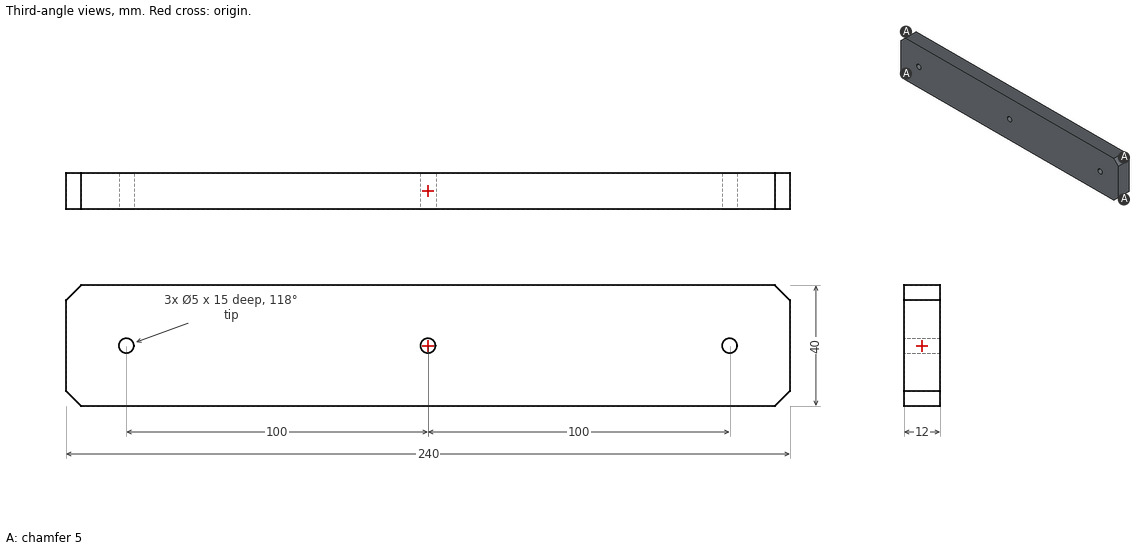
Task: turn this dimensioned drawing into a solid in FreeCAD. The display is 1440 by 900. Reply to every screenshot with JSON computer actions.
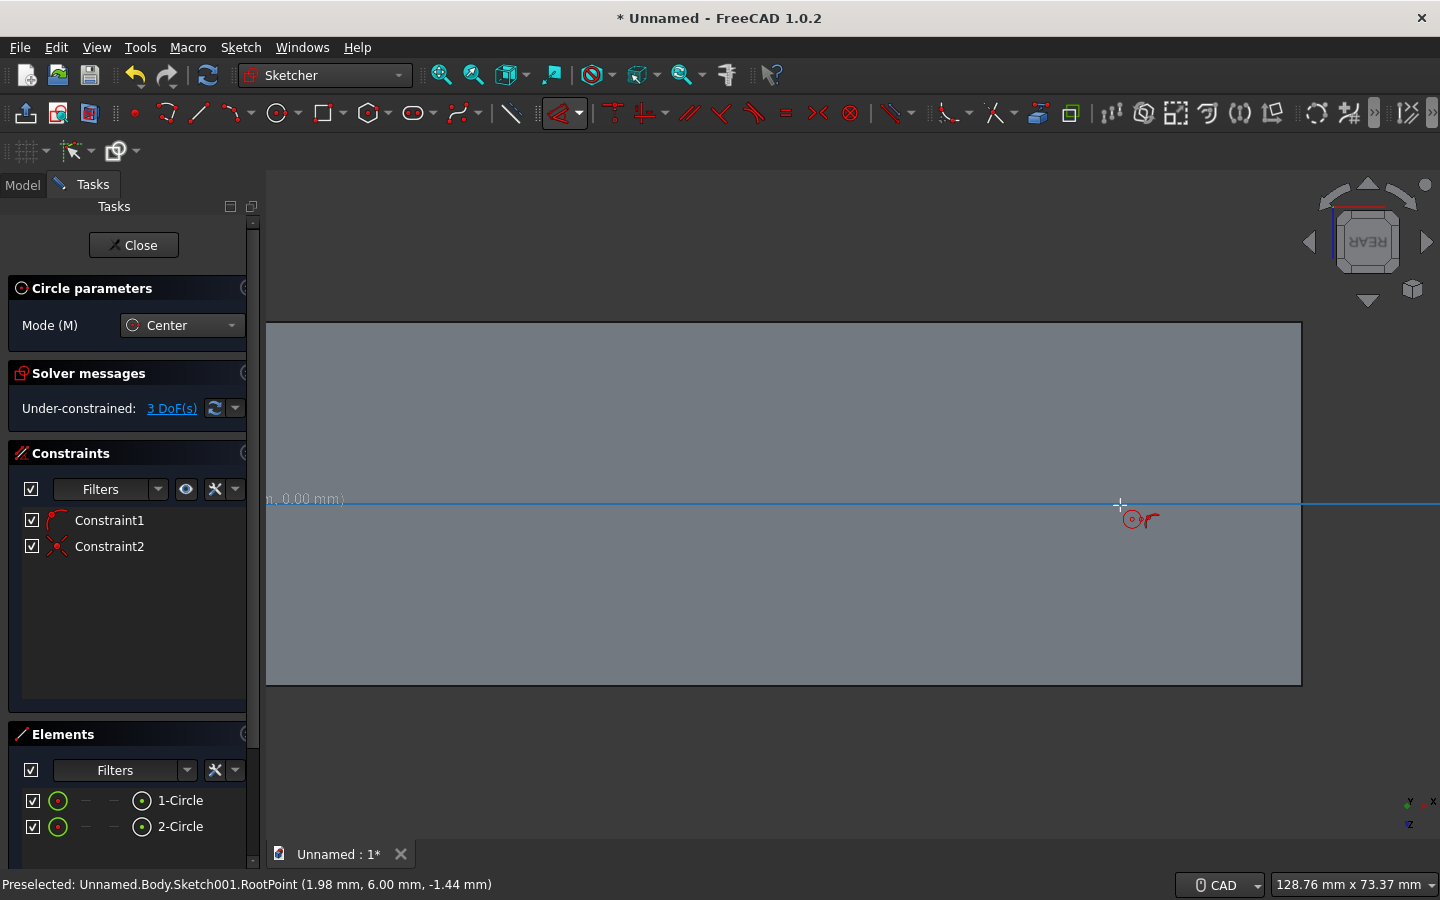
{"action": "left_click", "coordinate": [1119, 504]}
{"action": "left_click", "coordinate": [1135, 488]}
{"action": "key", "text": "Escape"}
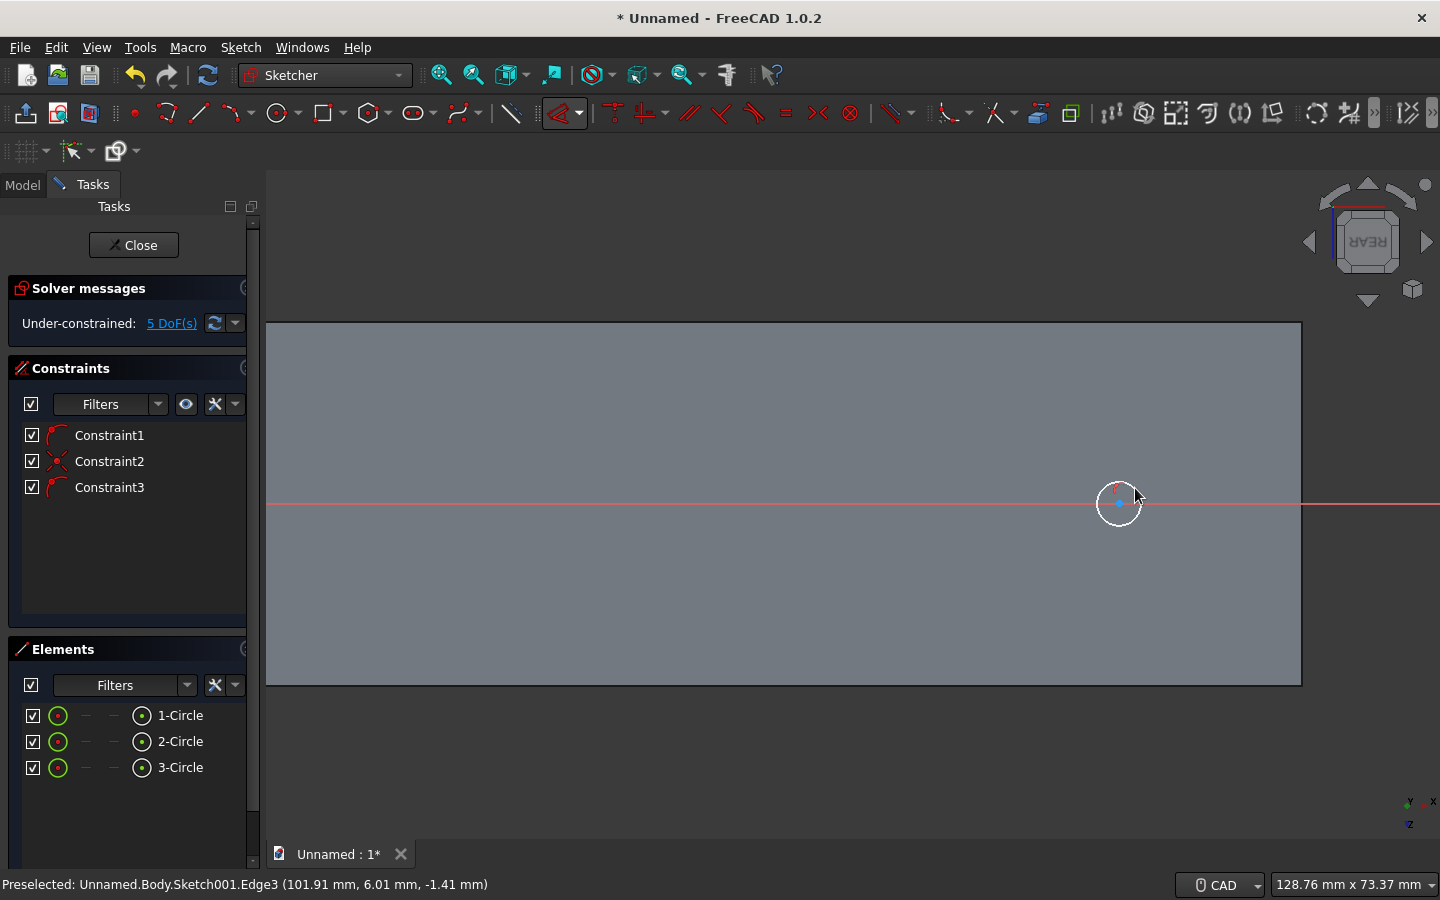
{"action": "scroll", "coordinate": [1120, 505], "scroll_direction": "down", "scroll_amount": 5}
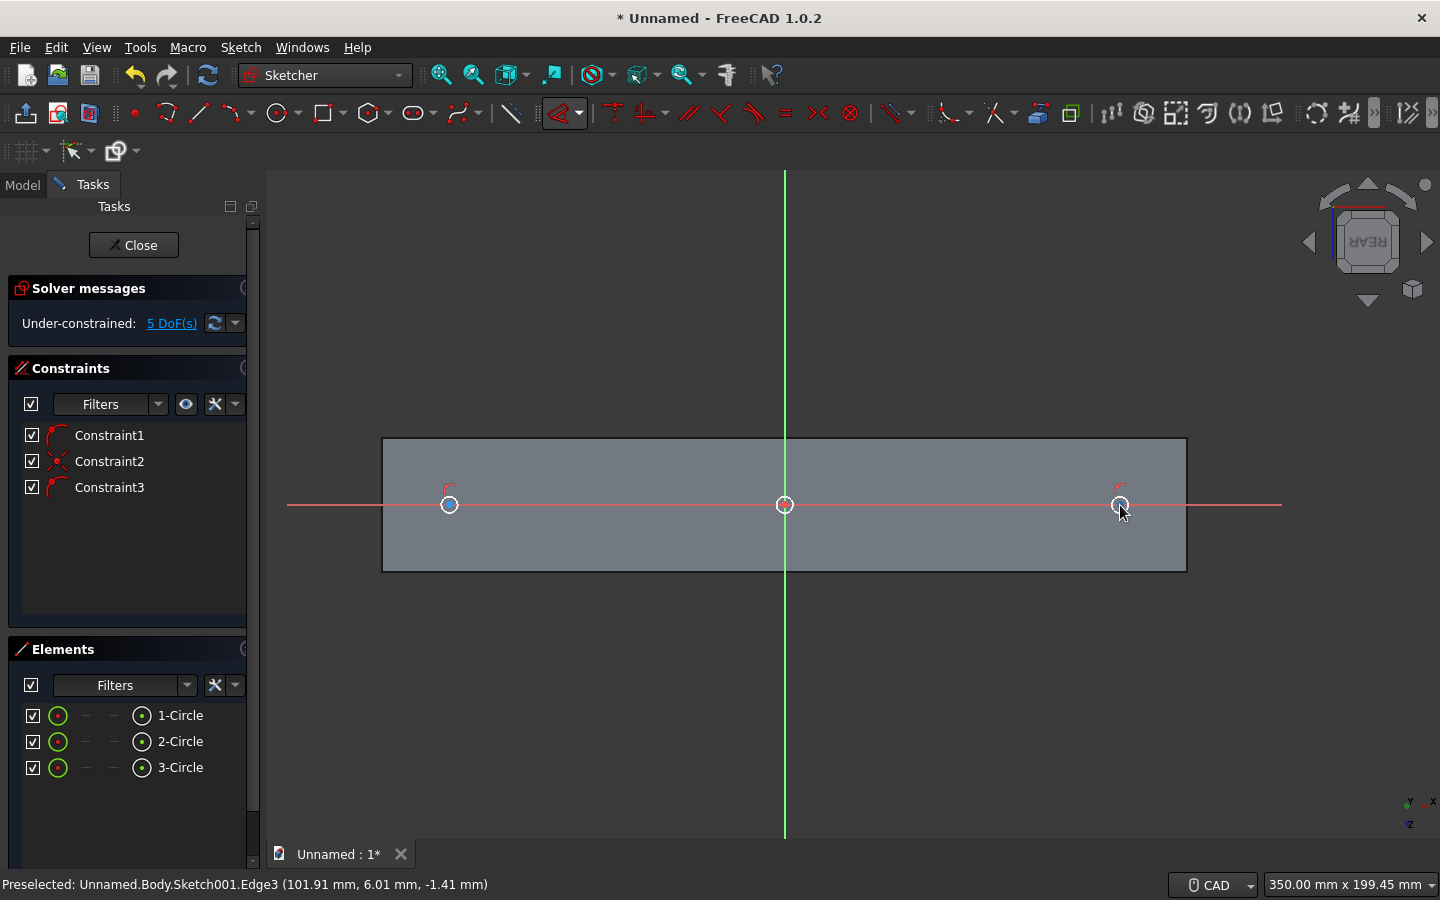
{"action": "scroll", "coordinate": [455, 499], "scroll_direction": "up", "scroll_amount": 5}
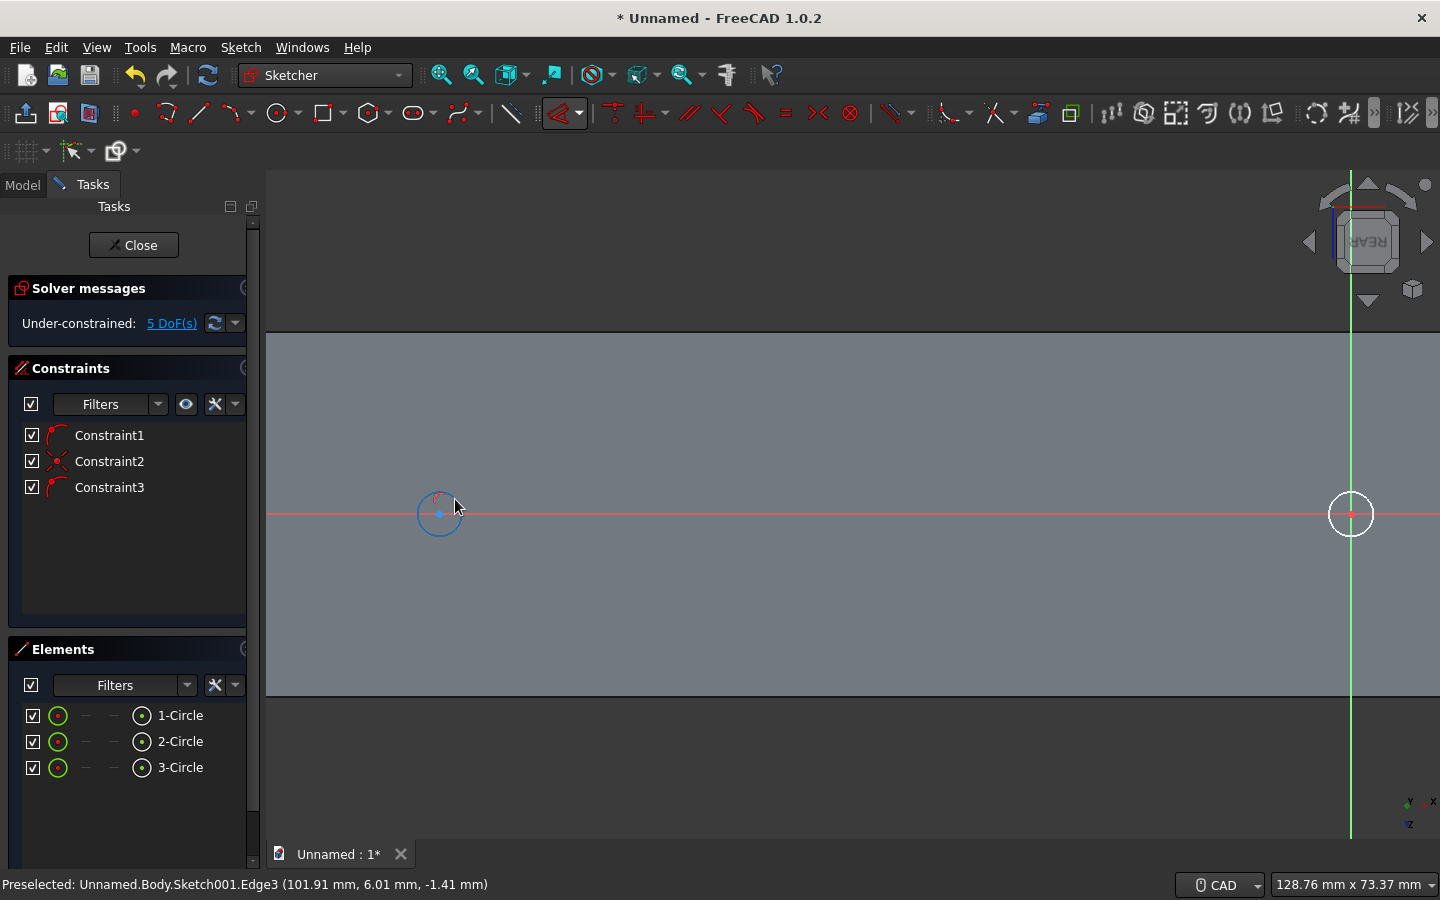
{"action": "left_click", "coordinate": [455, 499]}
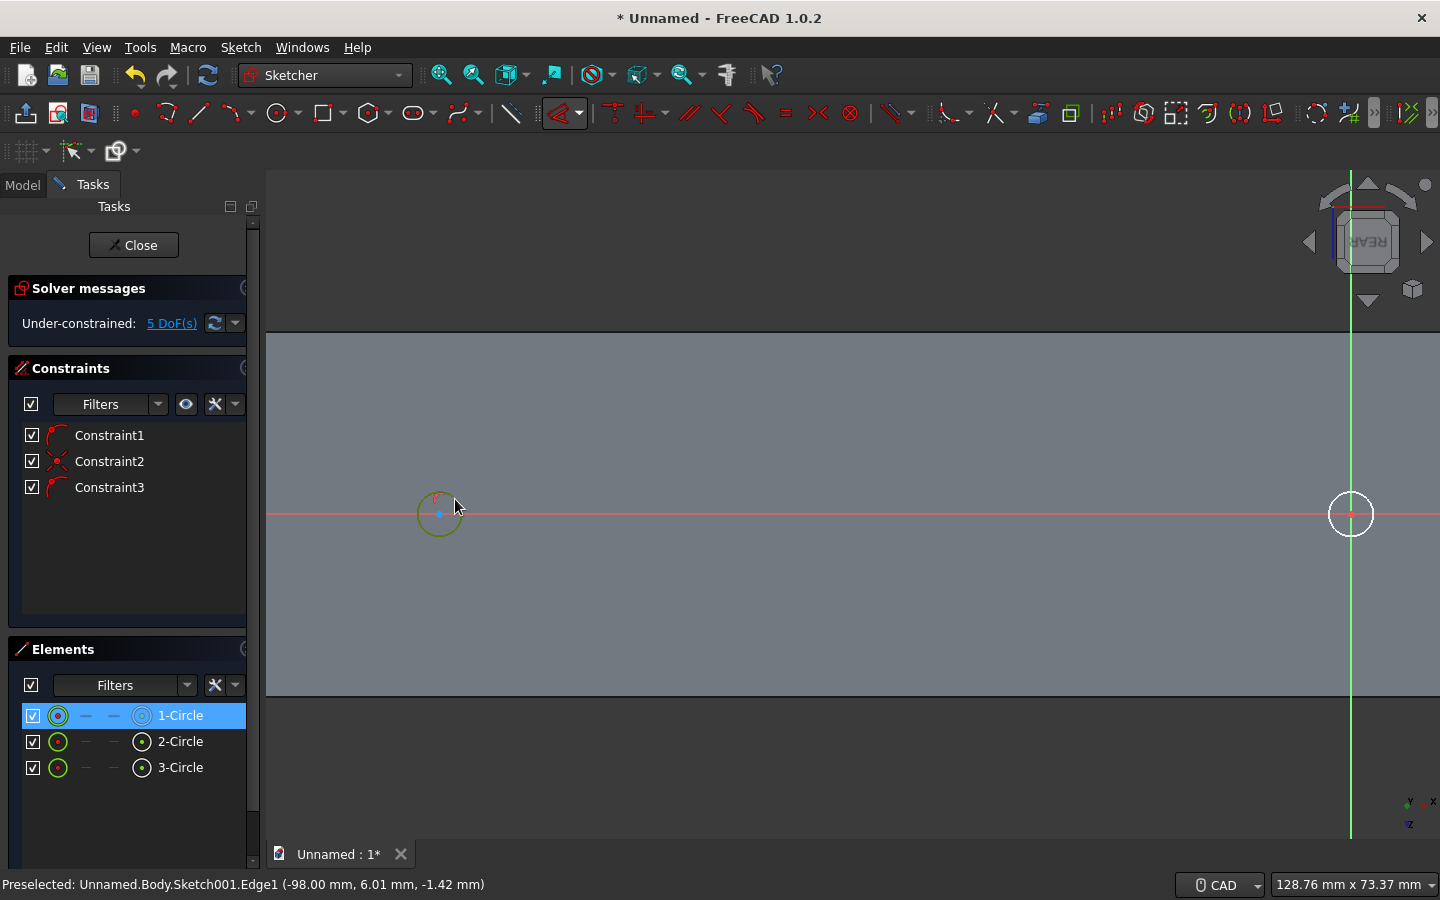
{"action": "scroll", "coordinate": [455, 499], "scroll_direction": "down", "scroll_amount": 5}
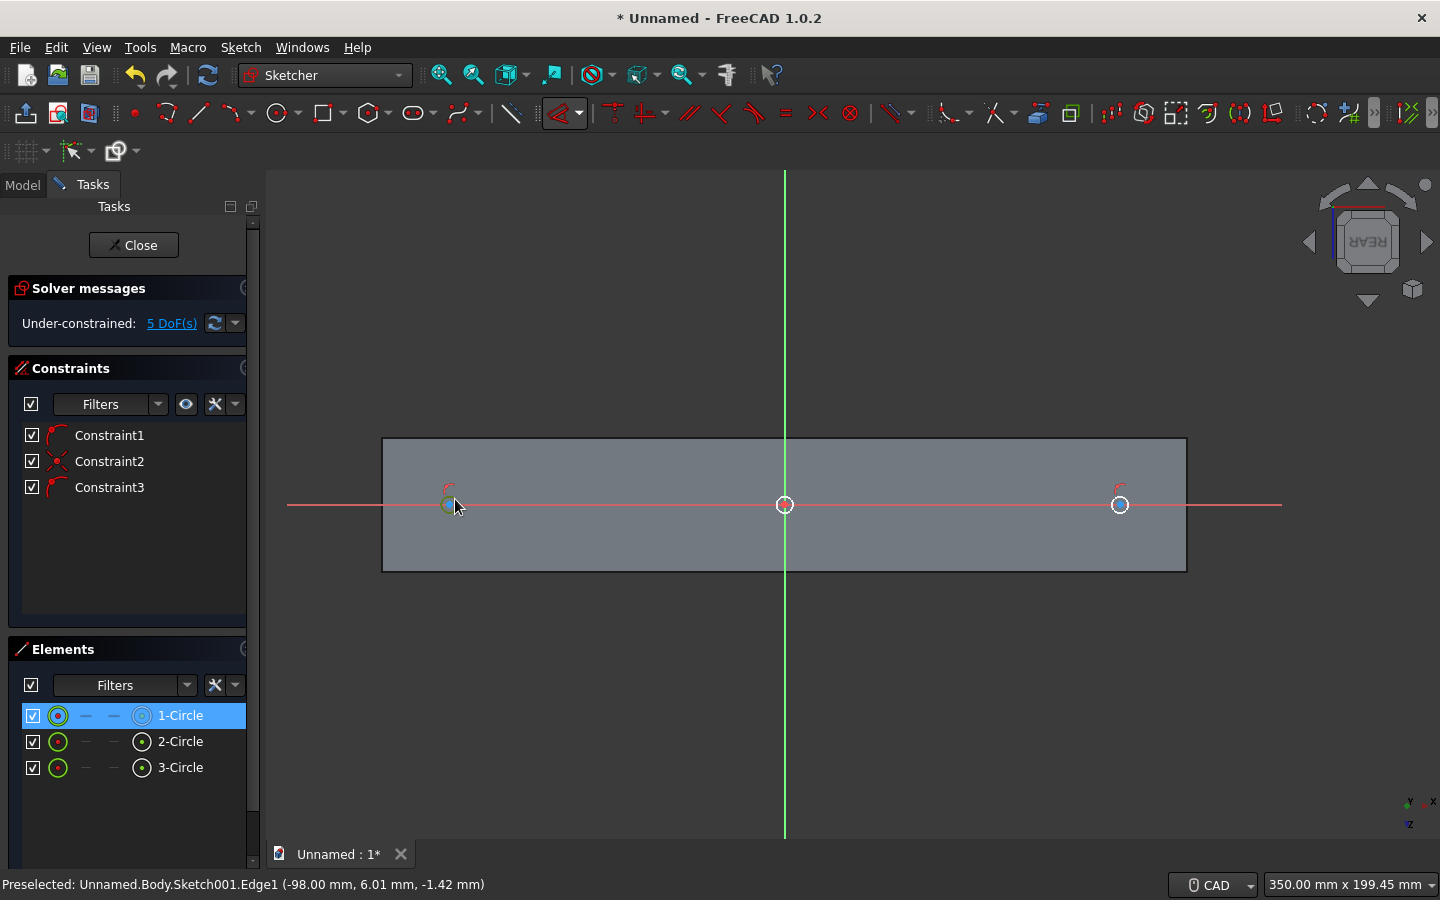
{"action": "scroll", "coordinate": [791, 499], "scroll_direction": "up", "scroll_amount": 5}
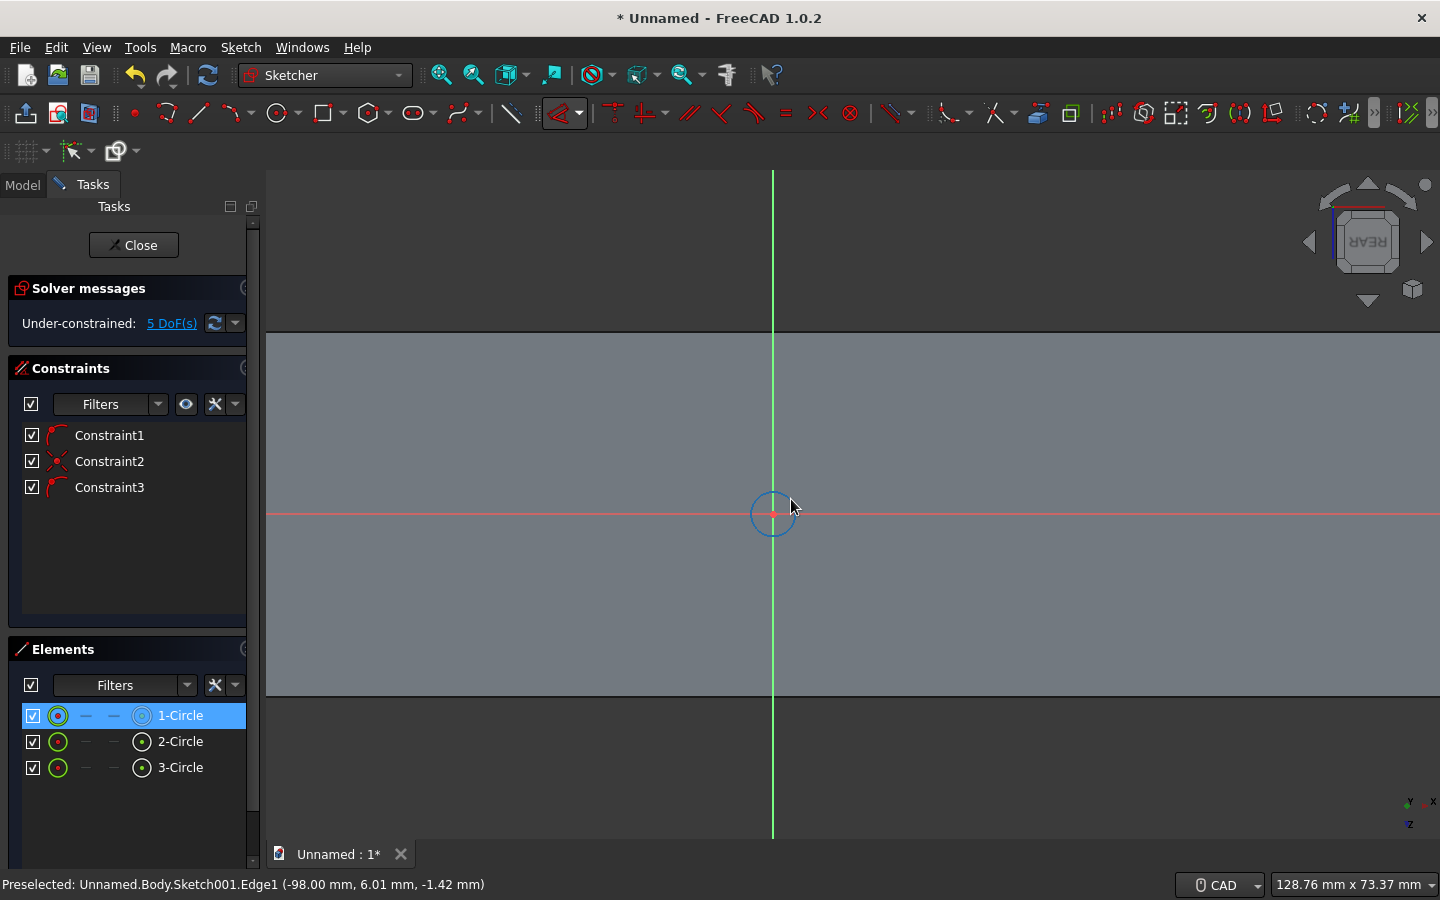
{"action": "left_click", "coordinate": [789, 499]}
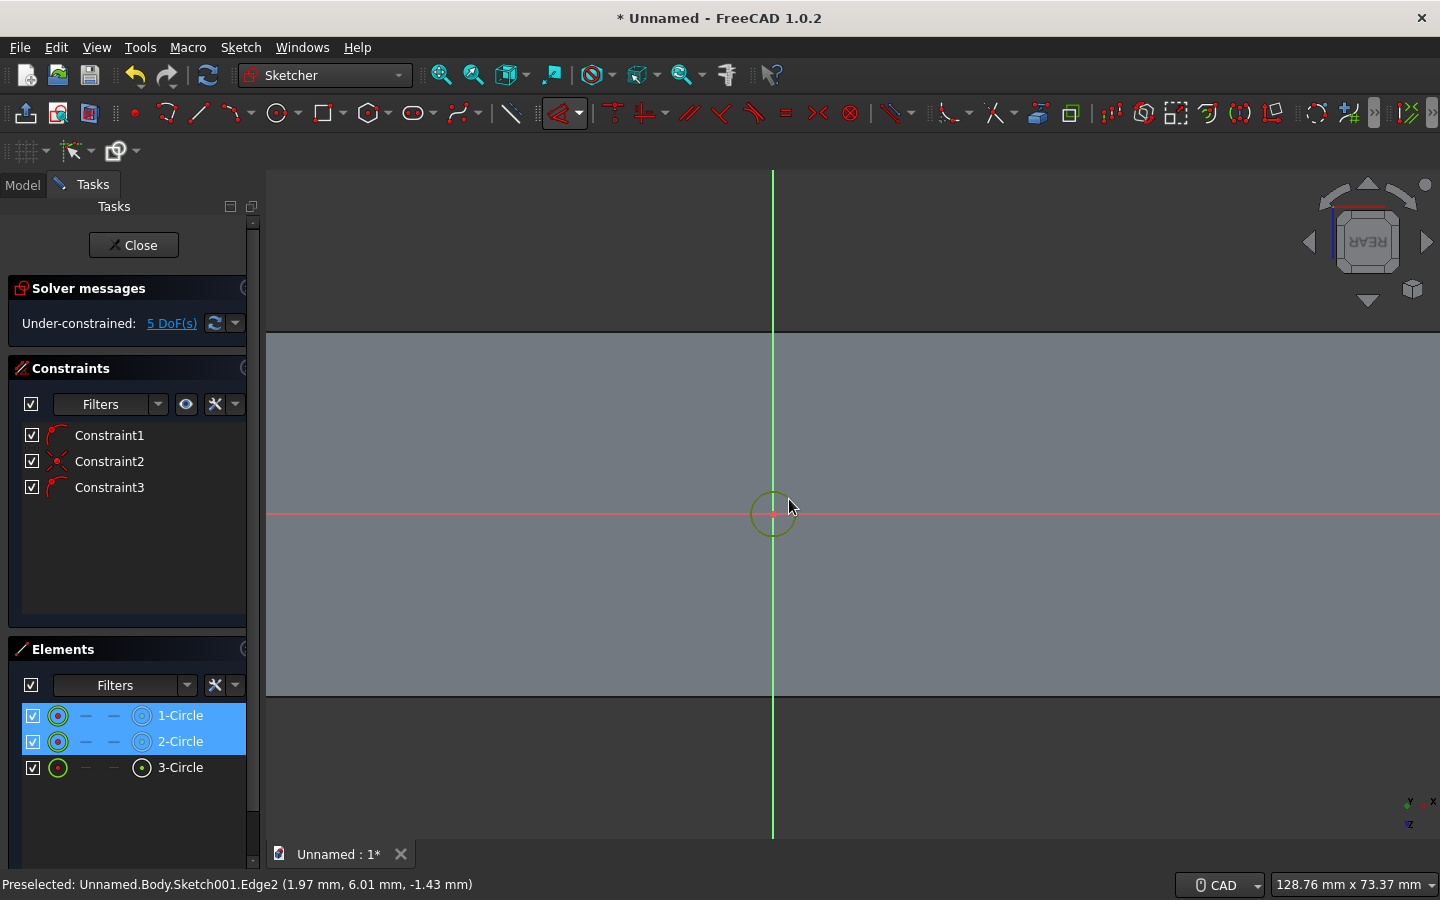
{"action": "scroll", "coordinate": [791, 499], "scroll_direction": "down", "scroll_amount": 5}